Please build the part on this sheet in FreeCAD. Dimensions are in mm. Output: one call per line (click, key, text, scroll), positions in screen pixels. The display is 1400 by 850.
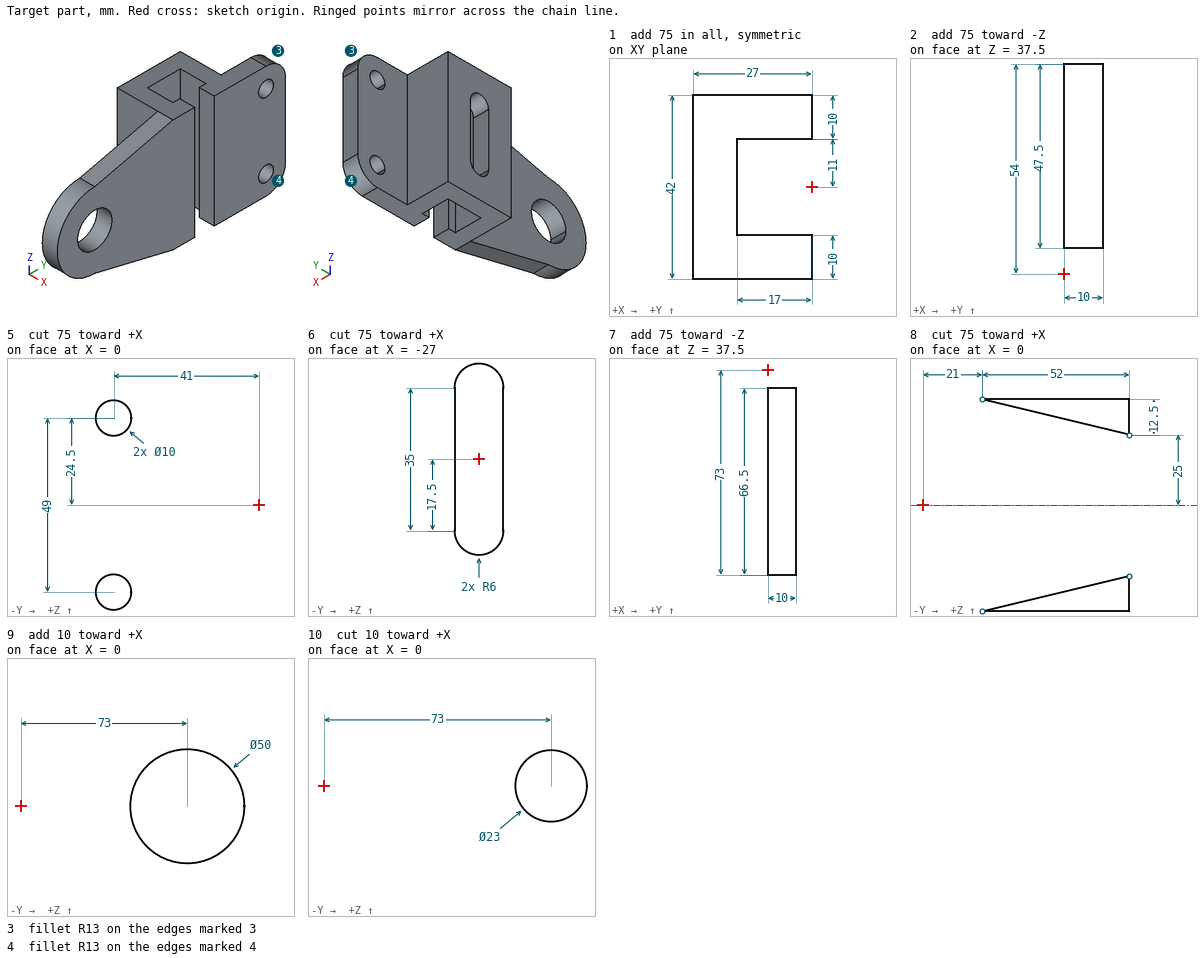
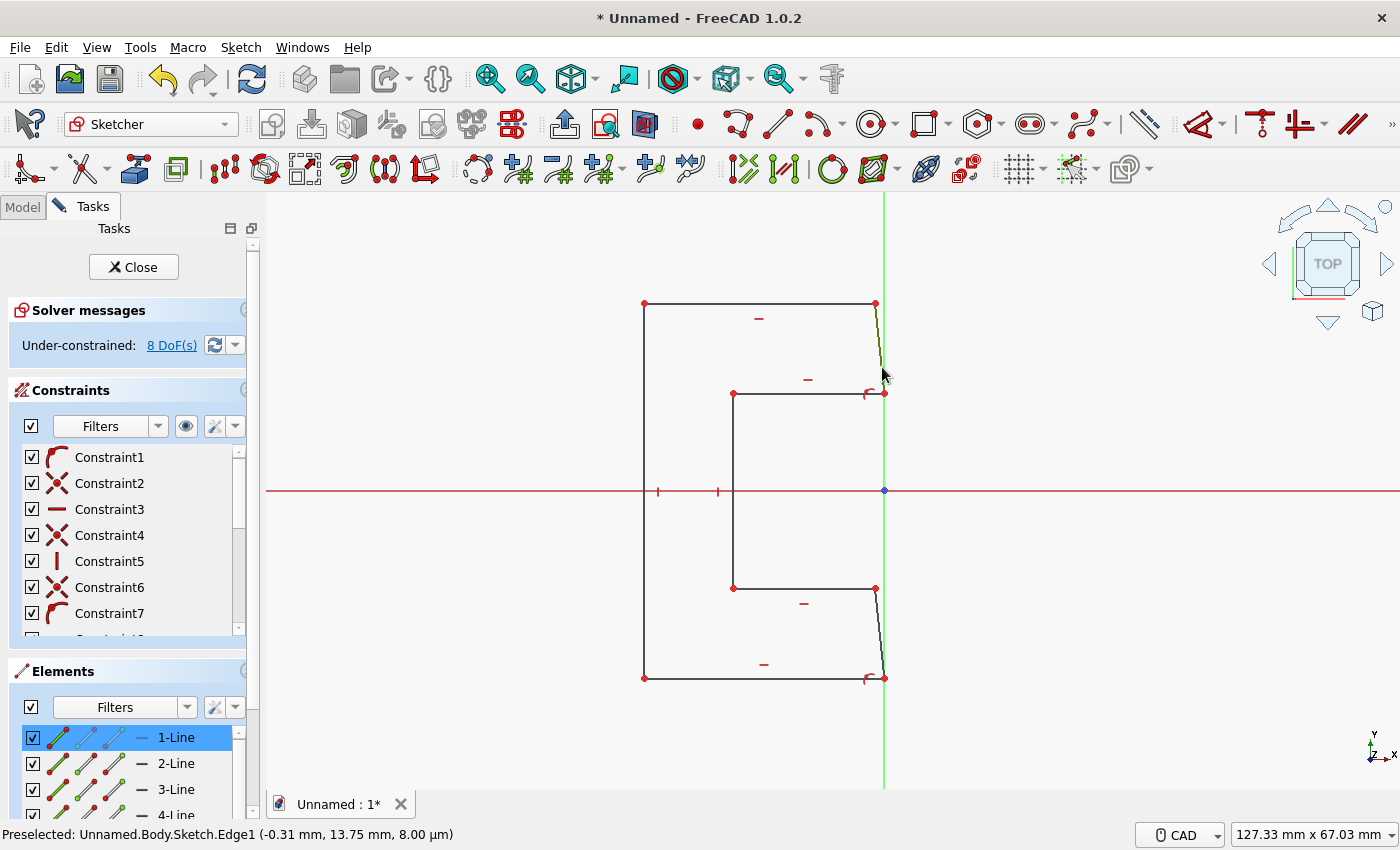
key(v)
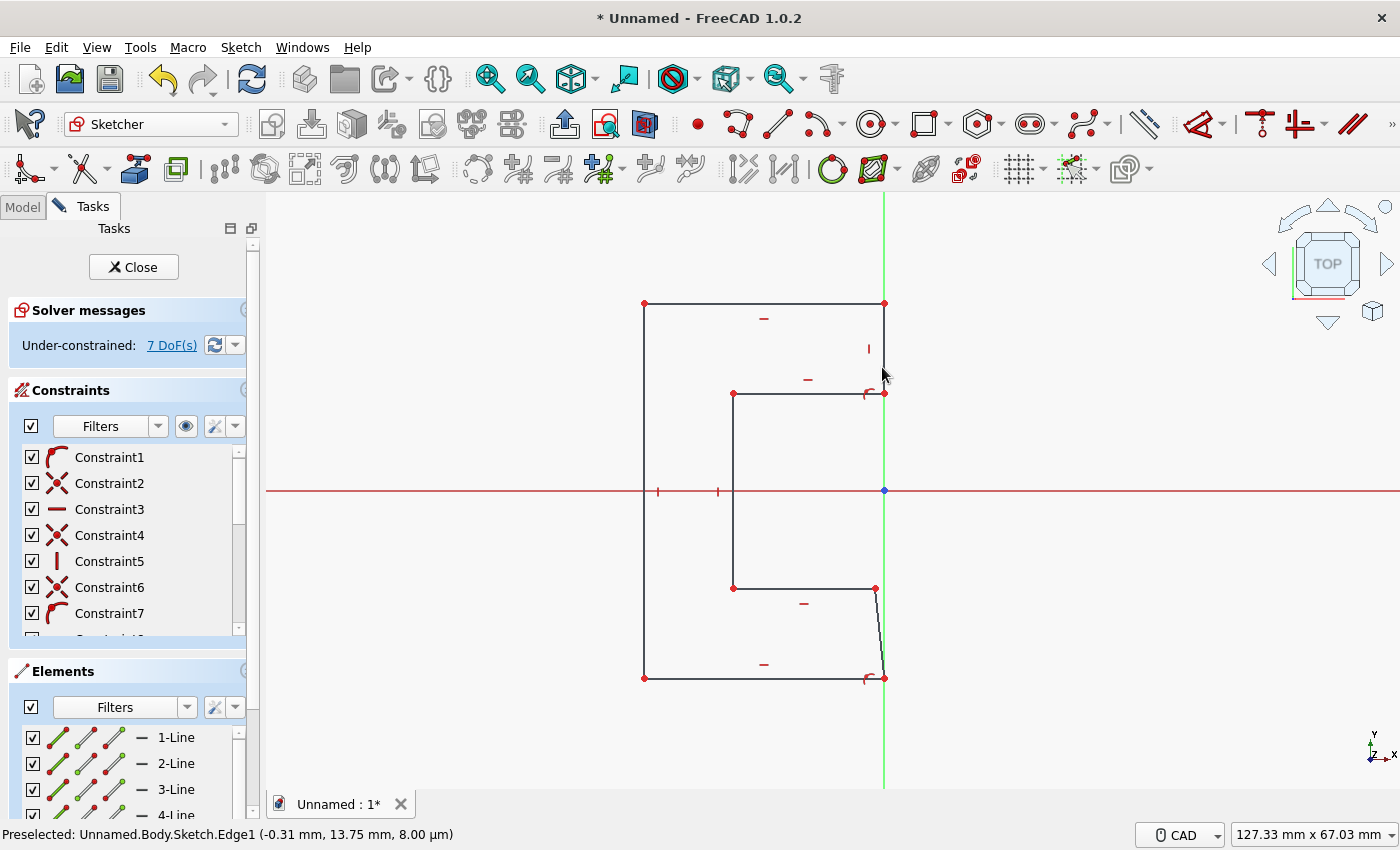
click(882, 652)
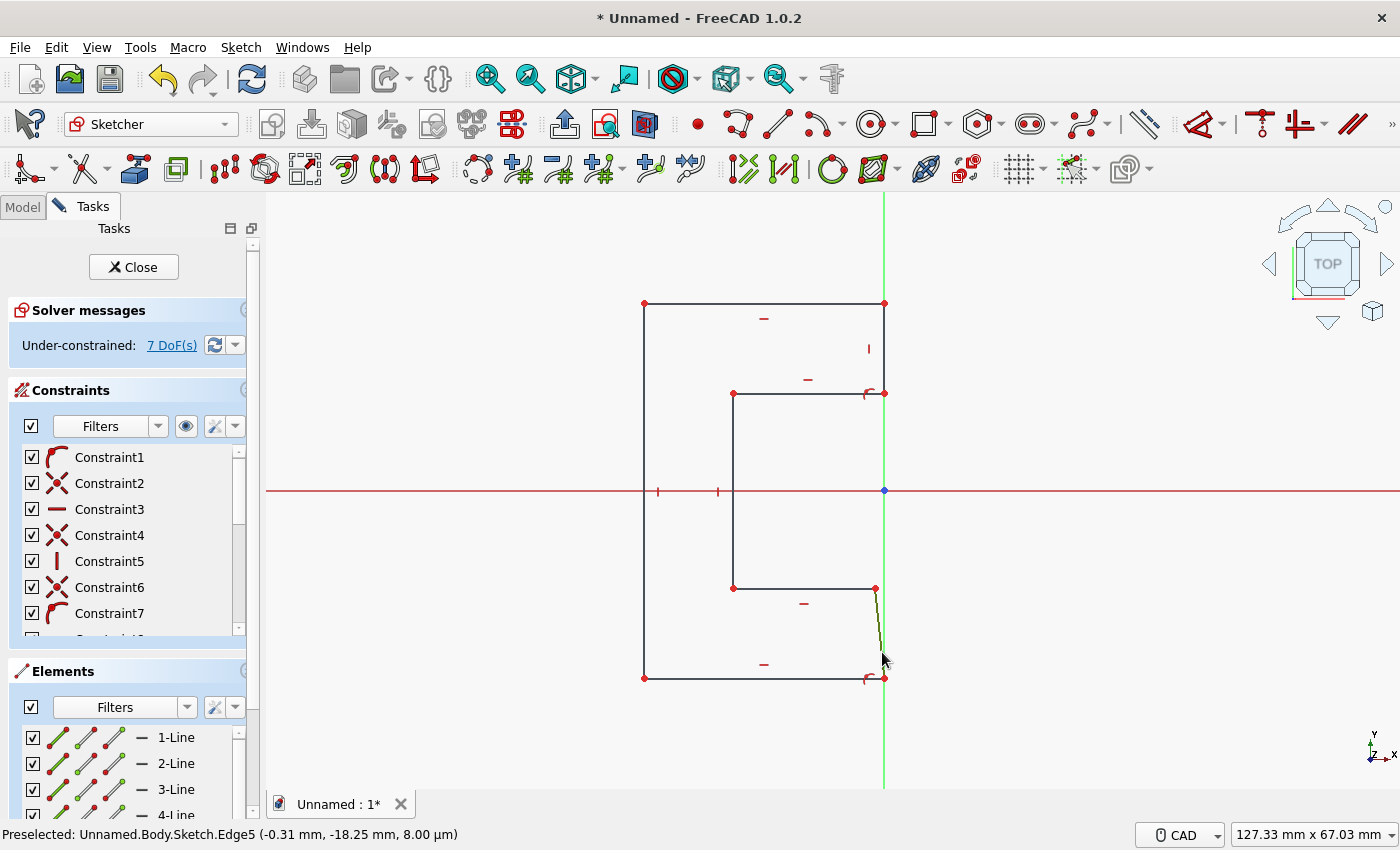
key(v)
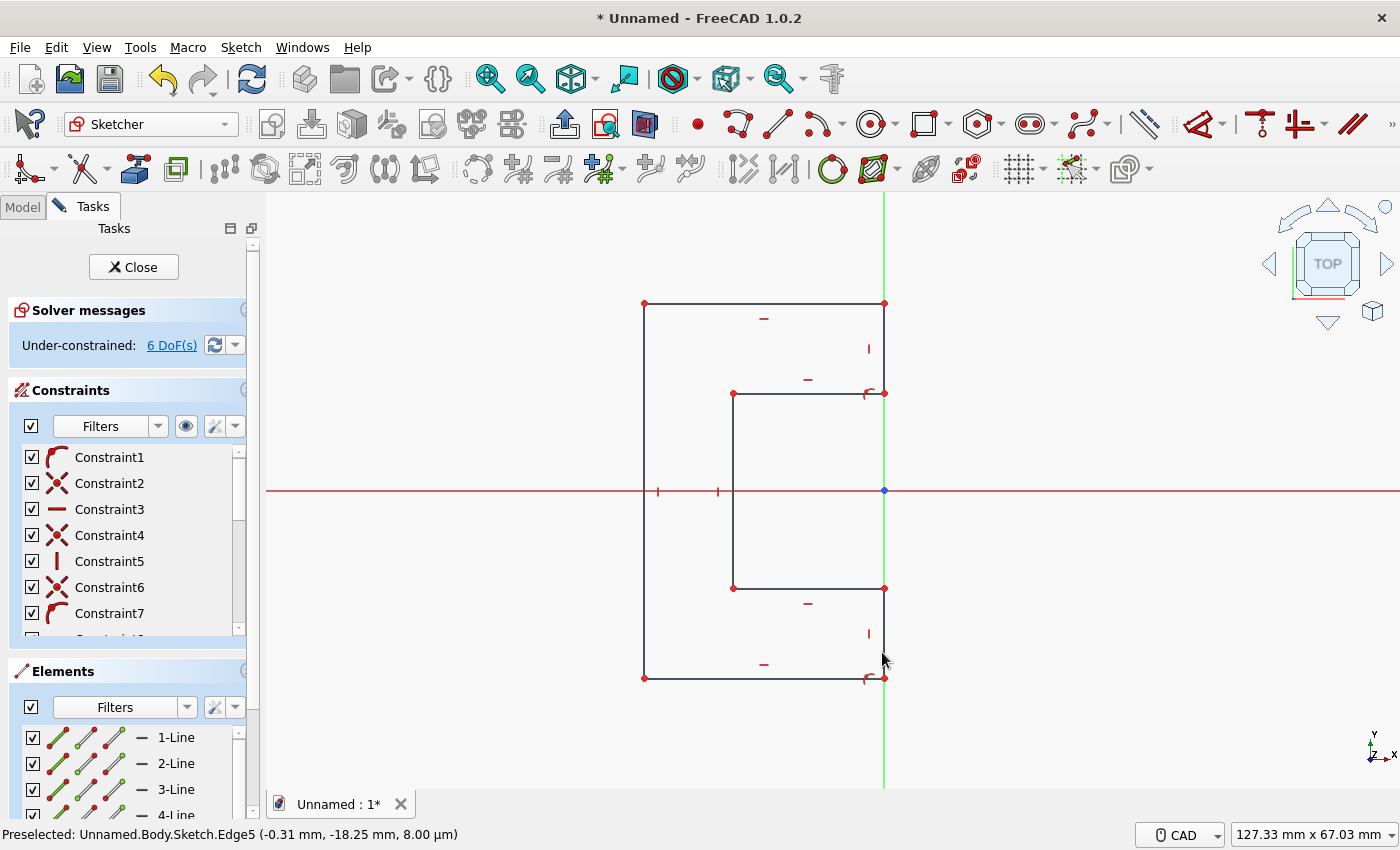
key(d)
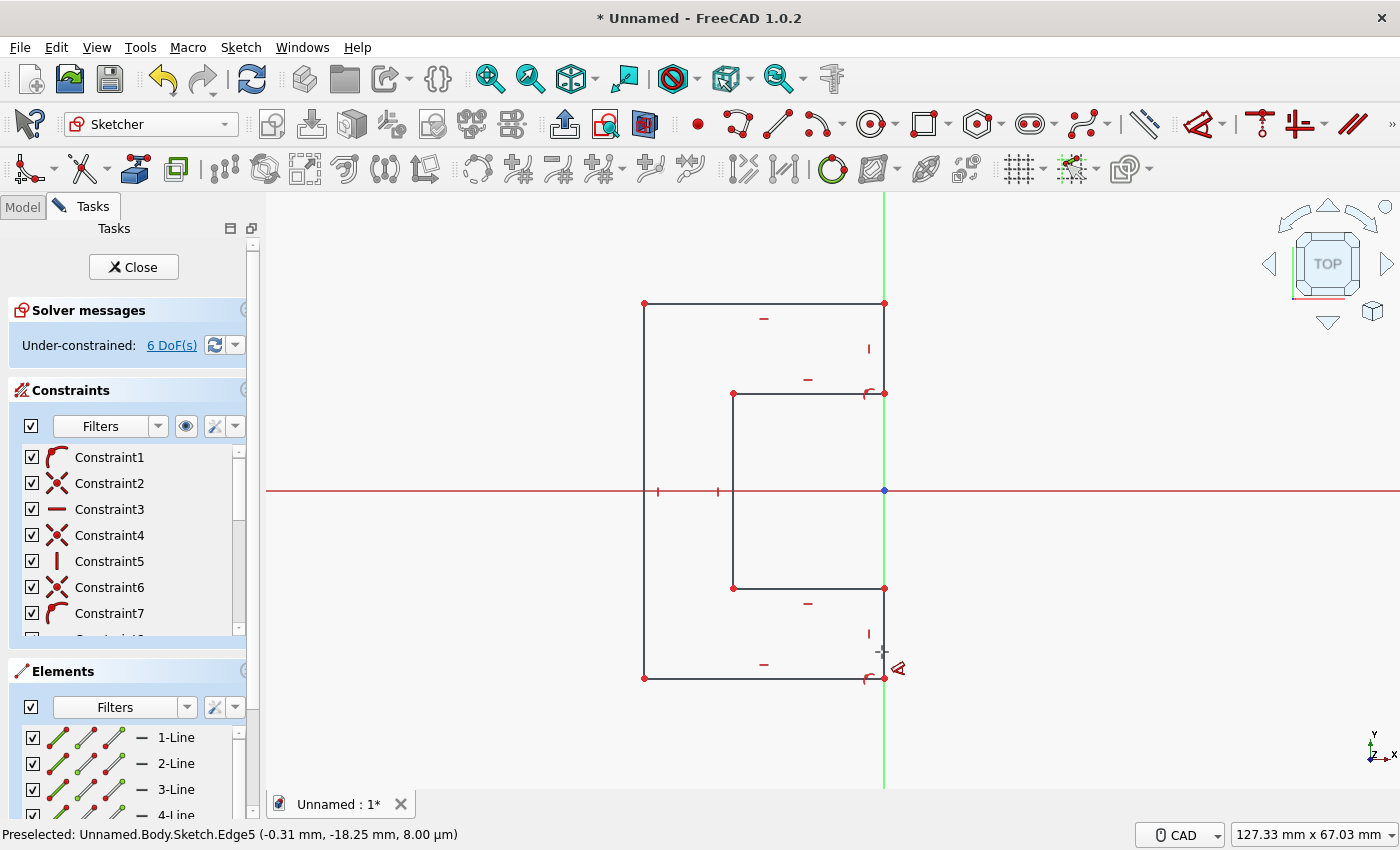
click(884, 367)
click(918, 349)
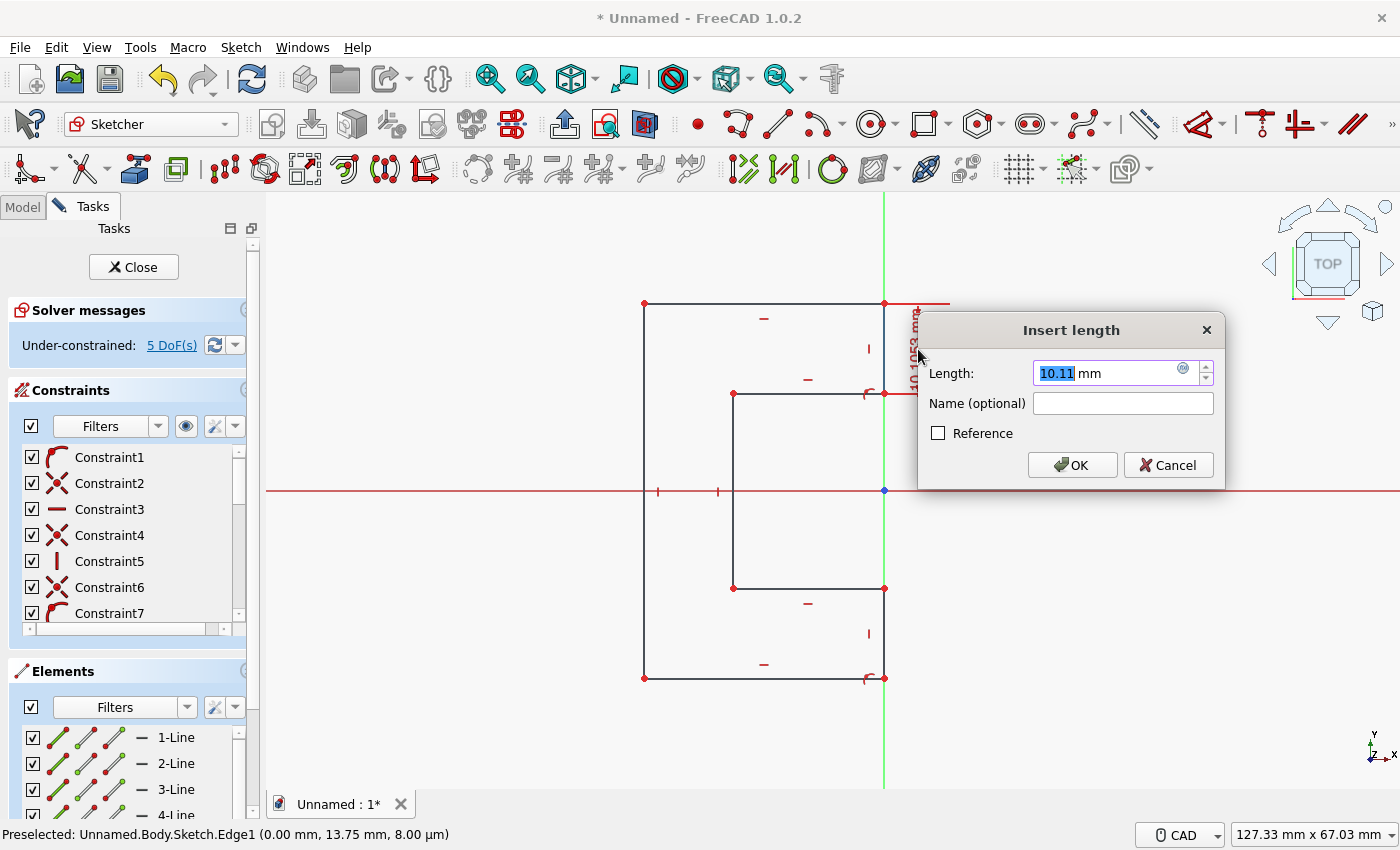
text(10)
key(Return)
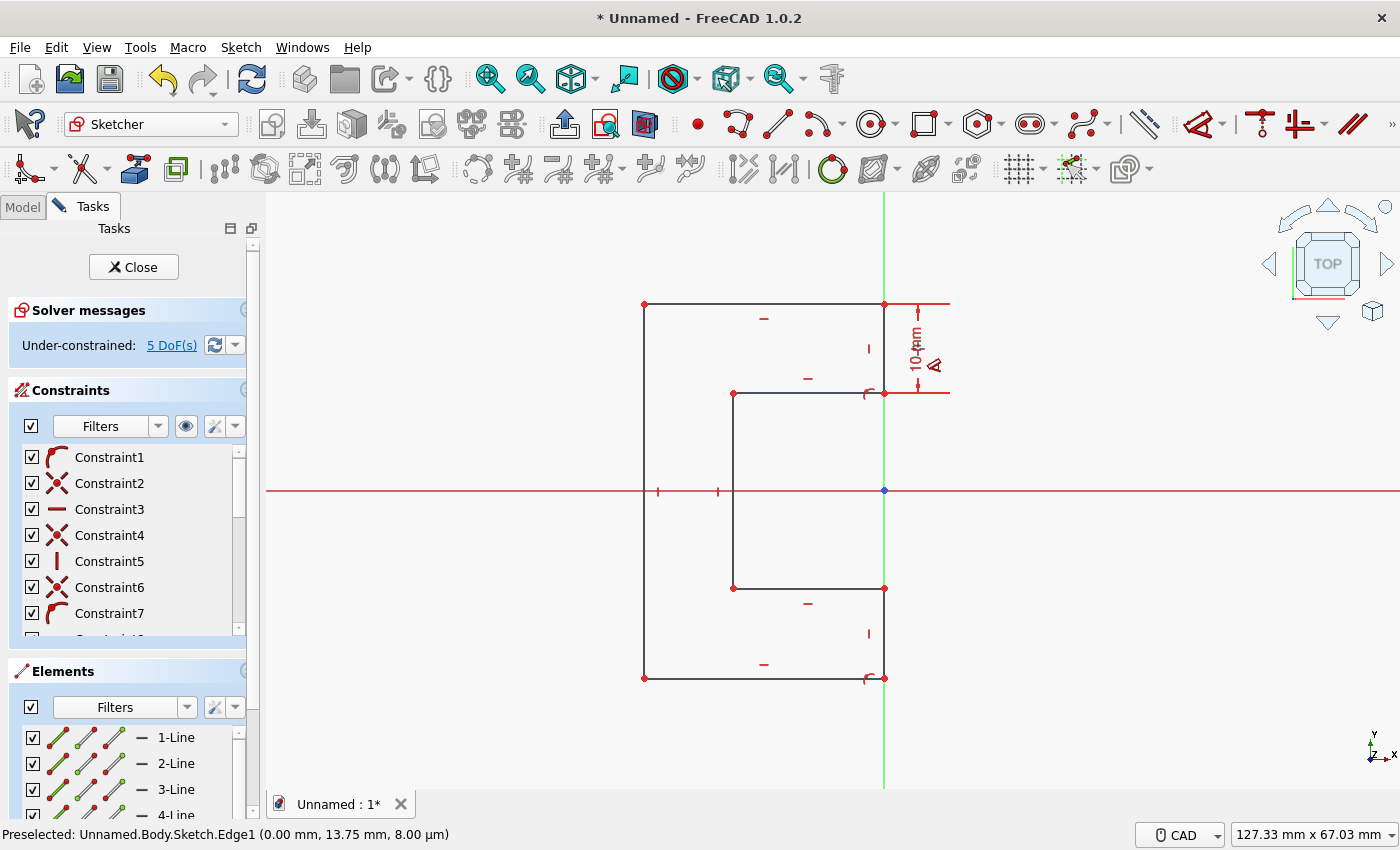
click(812, 304)
click(764, 270)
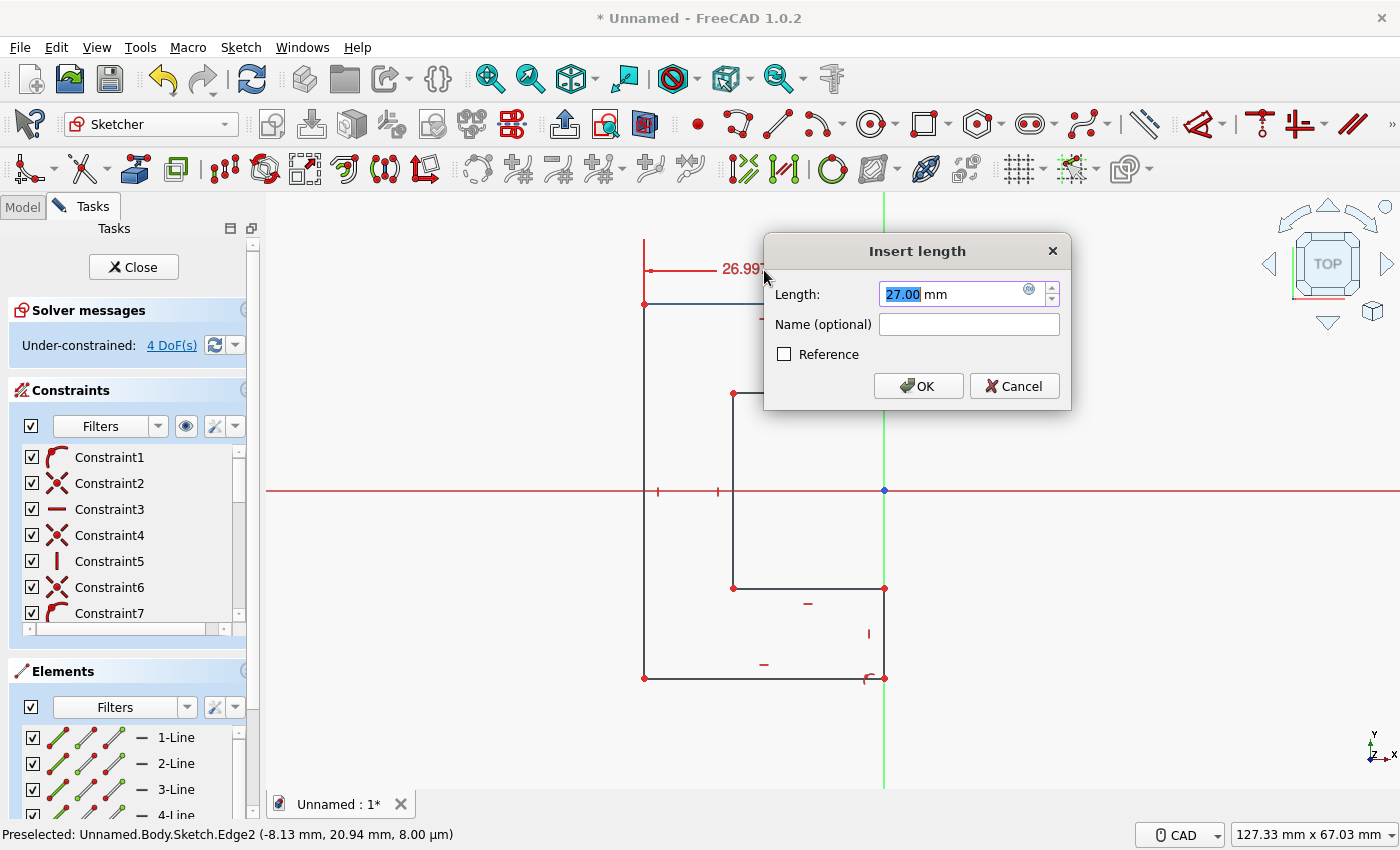
text(27)
key(Return)